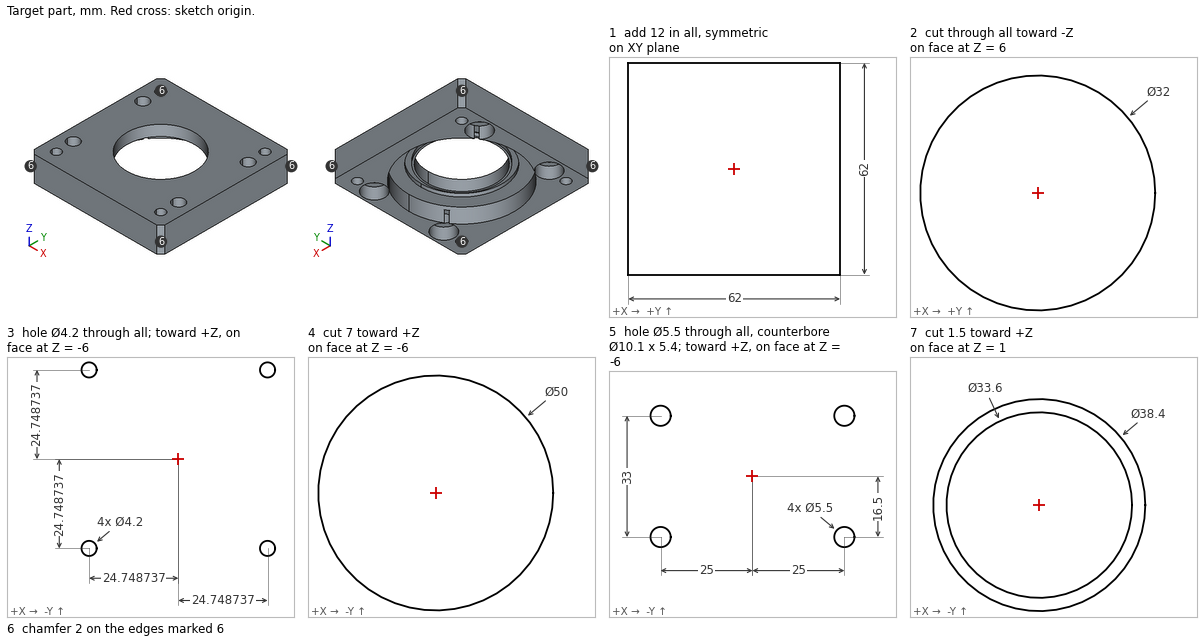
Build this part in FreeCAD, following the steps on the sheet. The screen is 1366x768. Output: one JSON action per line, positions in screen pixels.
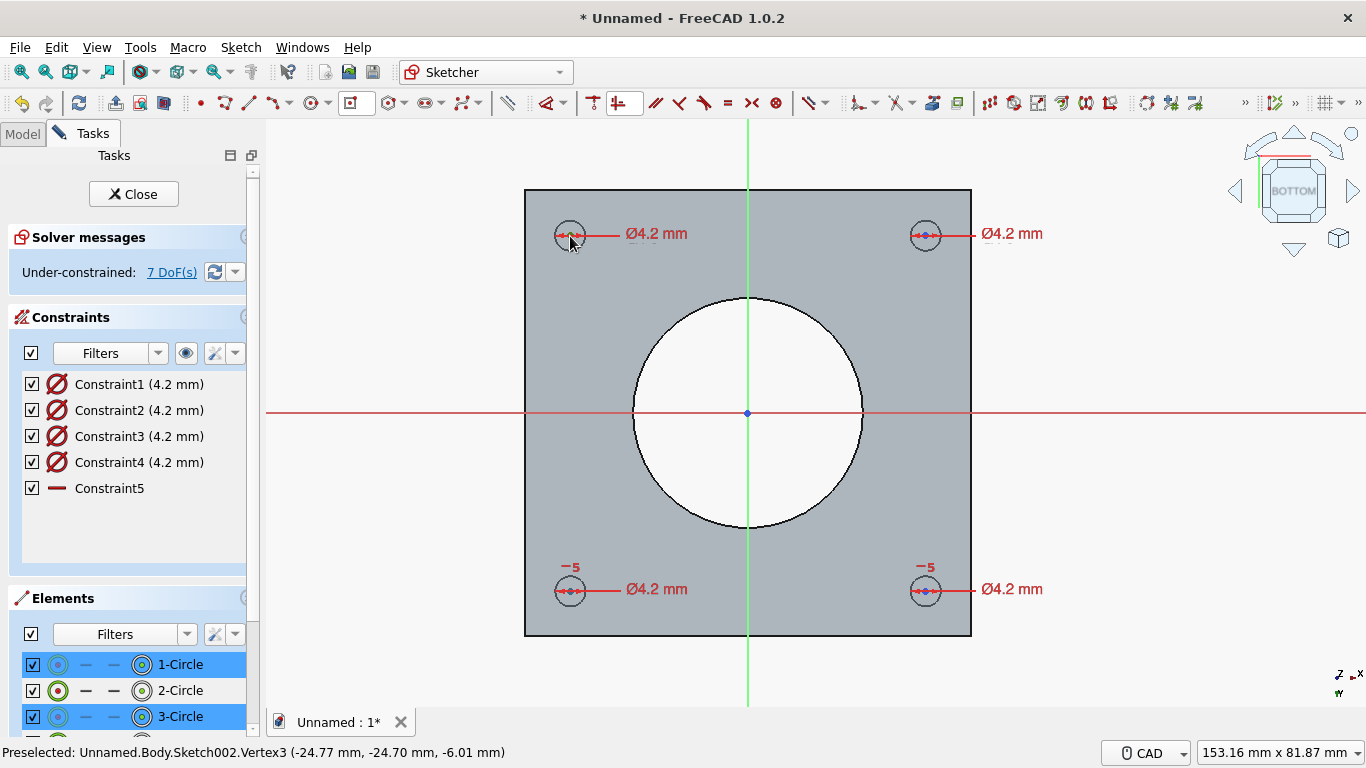
{"action": "left_click", "coordinate": [638, 104]}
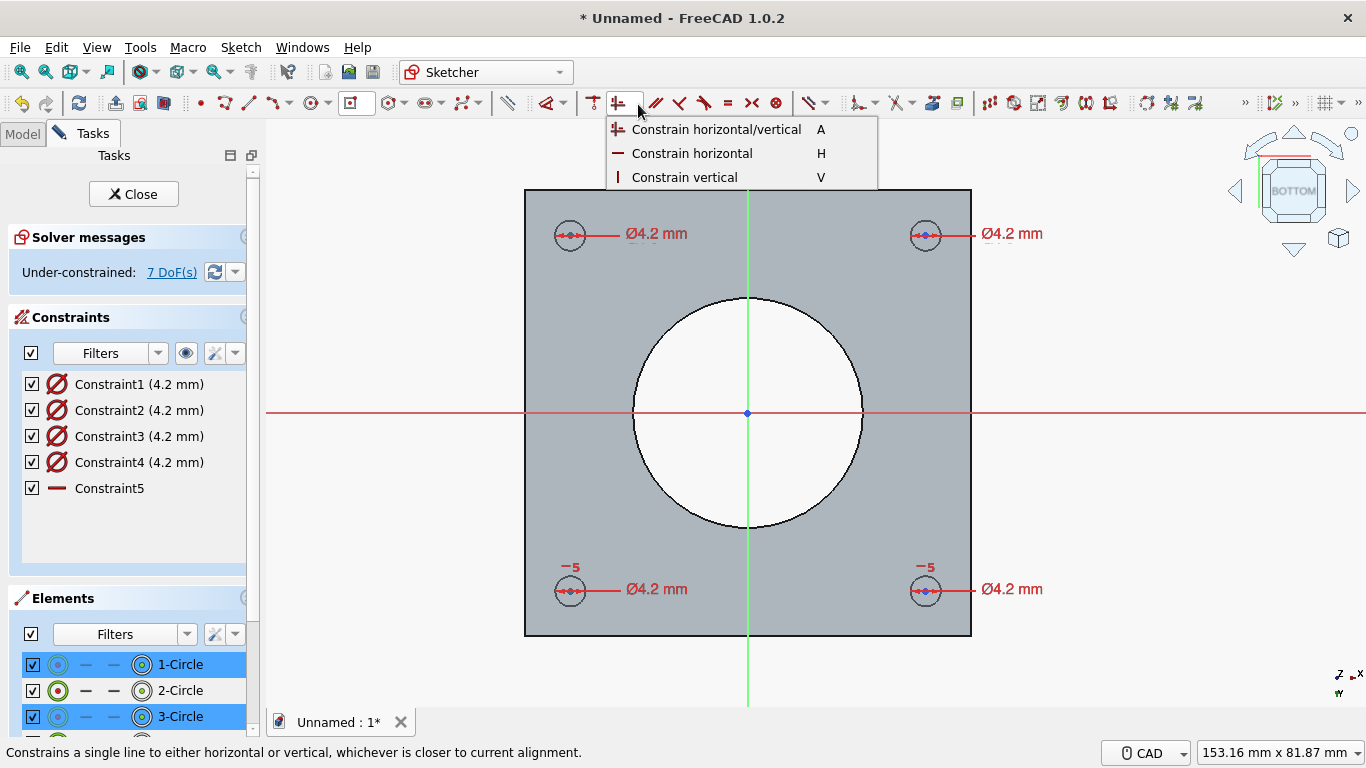
{"action": "left_click", "coordinate": [742, 177]}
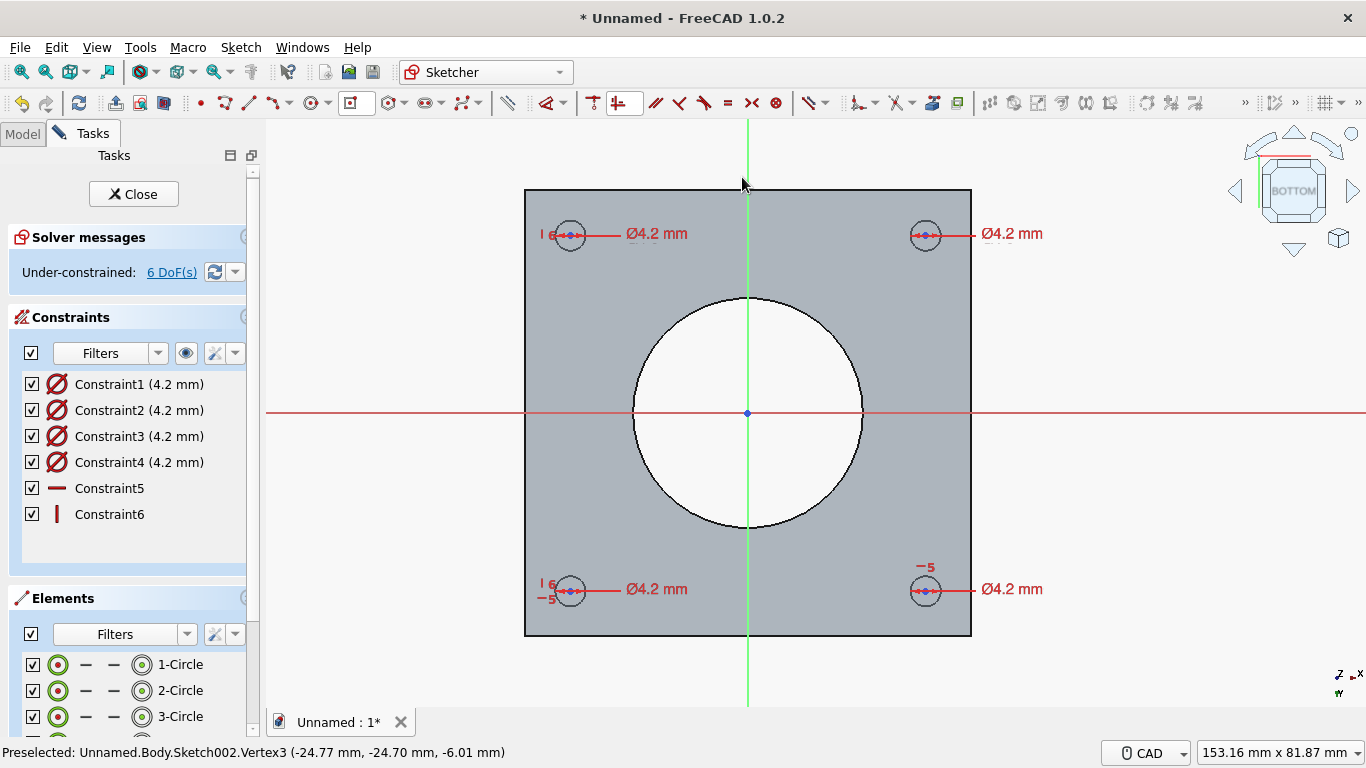
{"action": "left_click", "coordinate": [926, 591]}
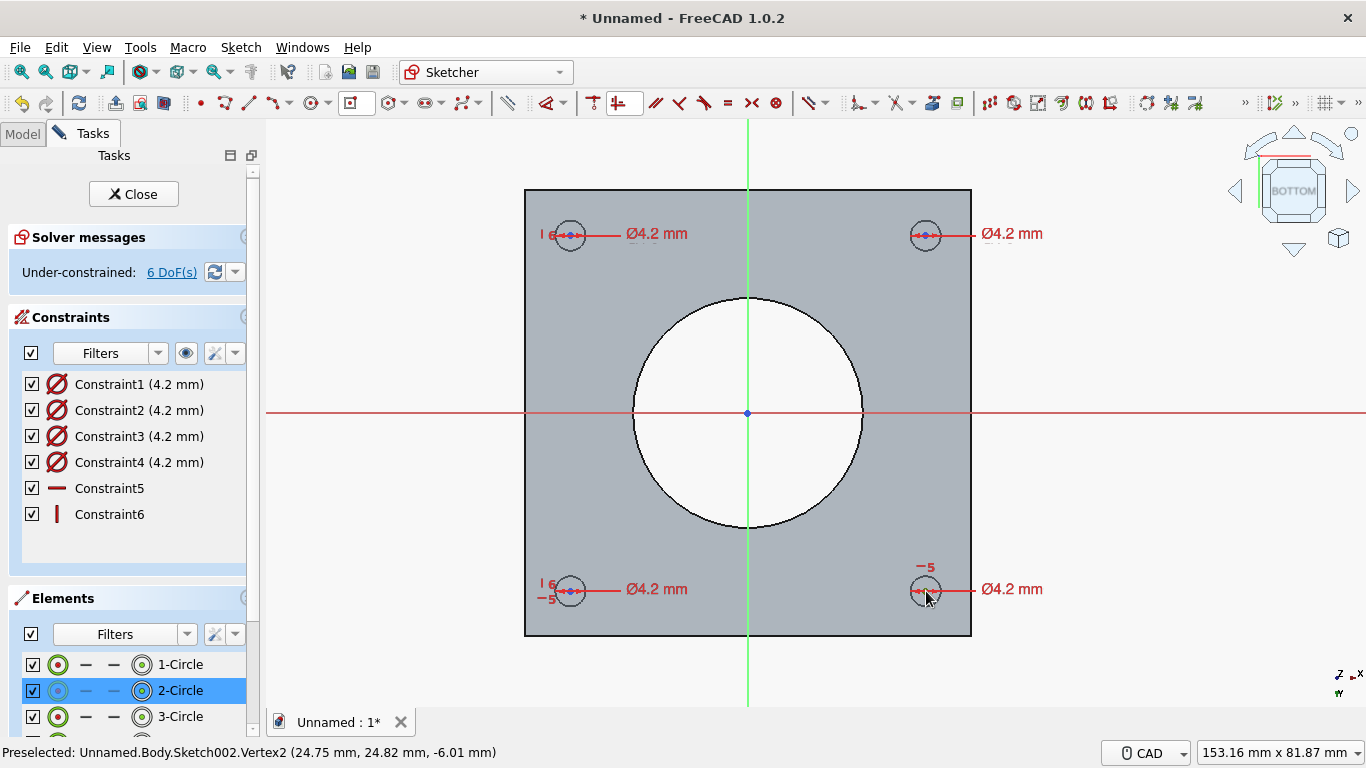
{"action": "left_click", "coordinate": [926, 236]}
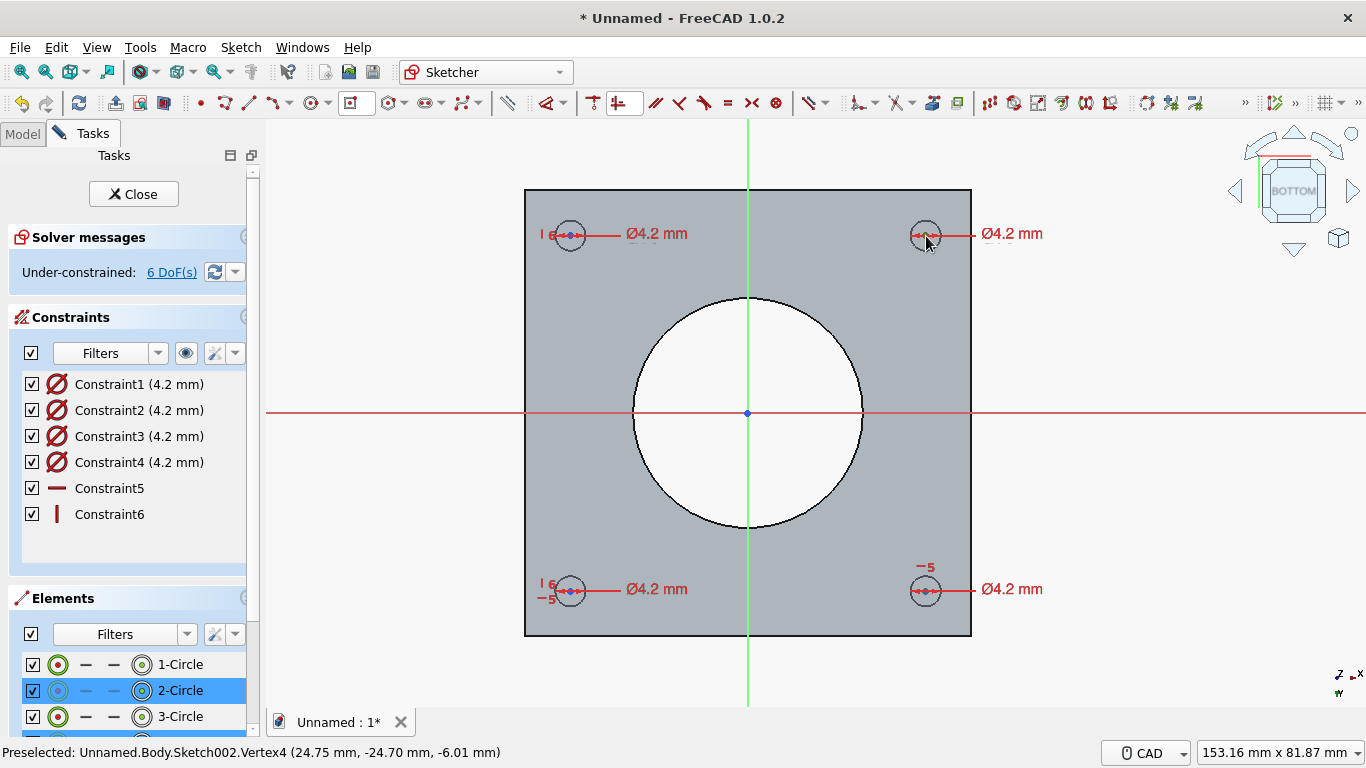
{"action": "left_click", "coordinate": [638, 104]}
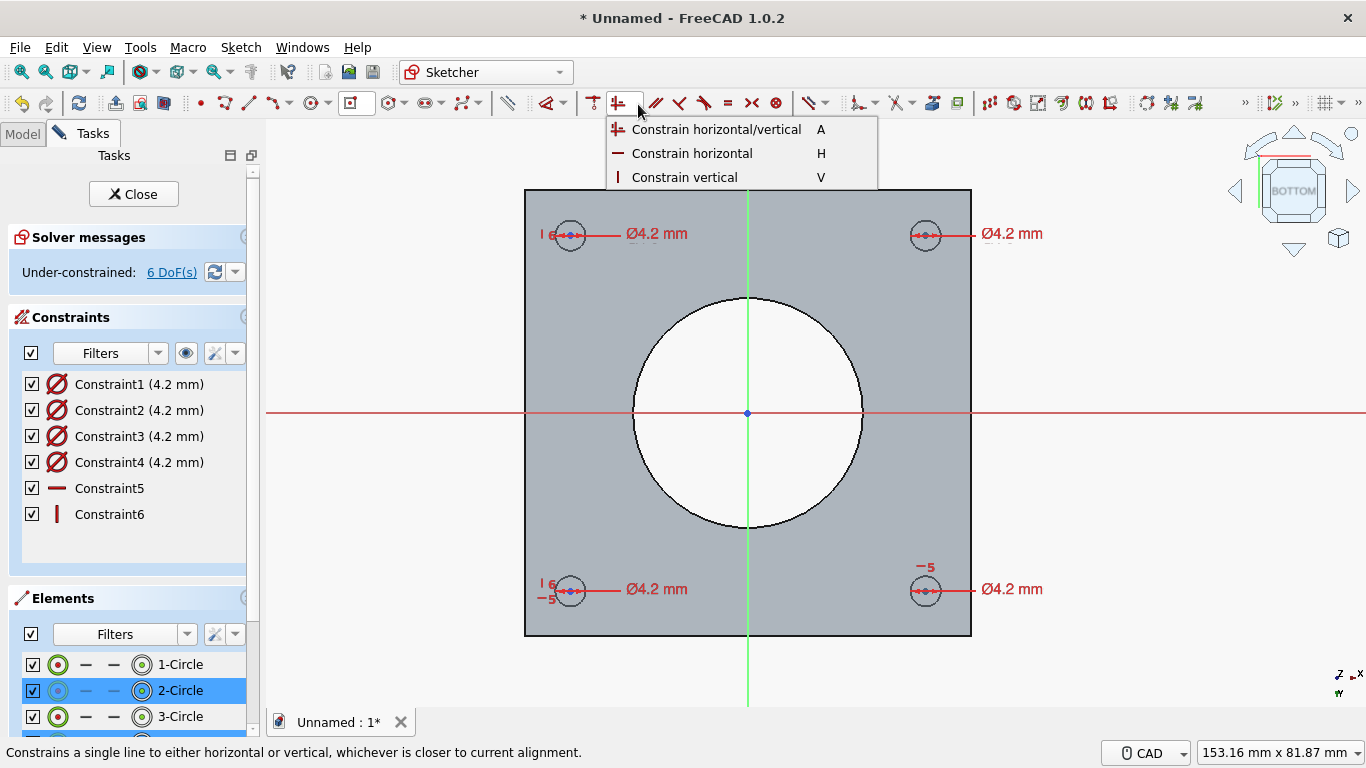
{"action": "left_click", "coordinate": [742, 177]}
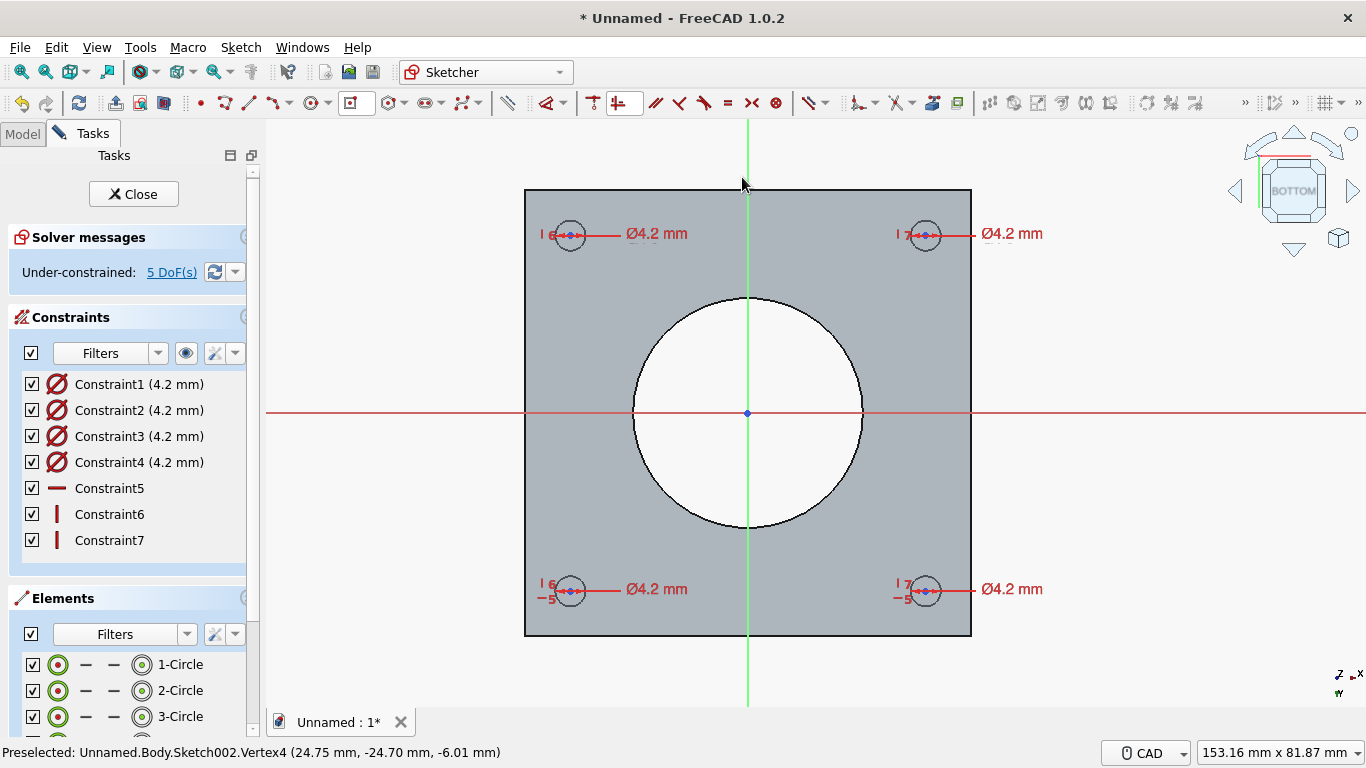
{"action": "left_click", "coordinate": [570, 236]}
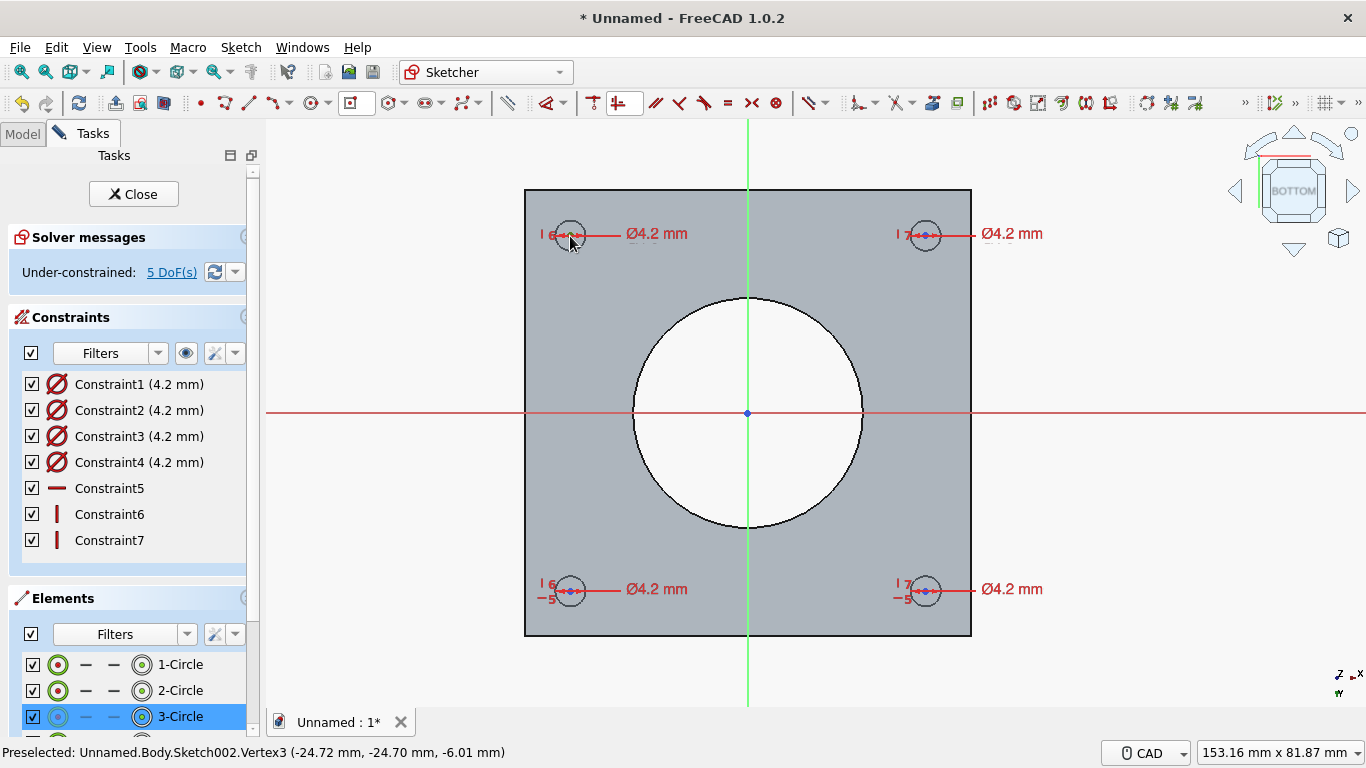
{"action": "left_click", "coordinate": [926, 236]}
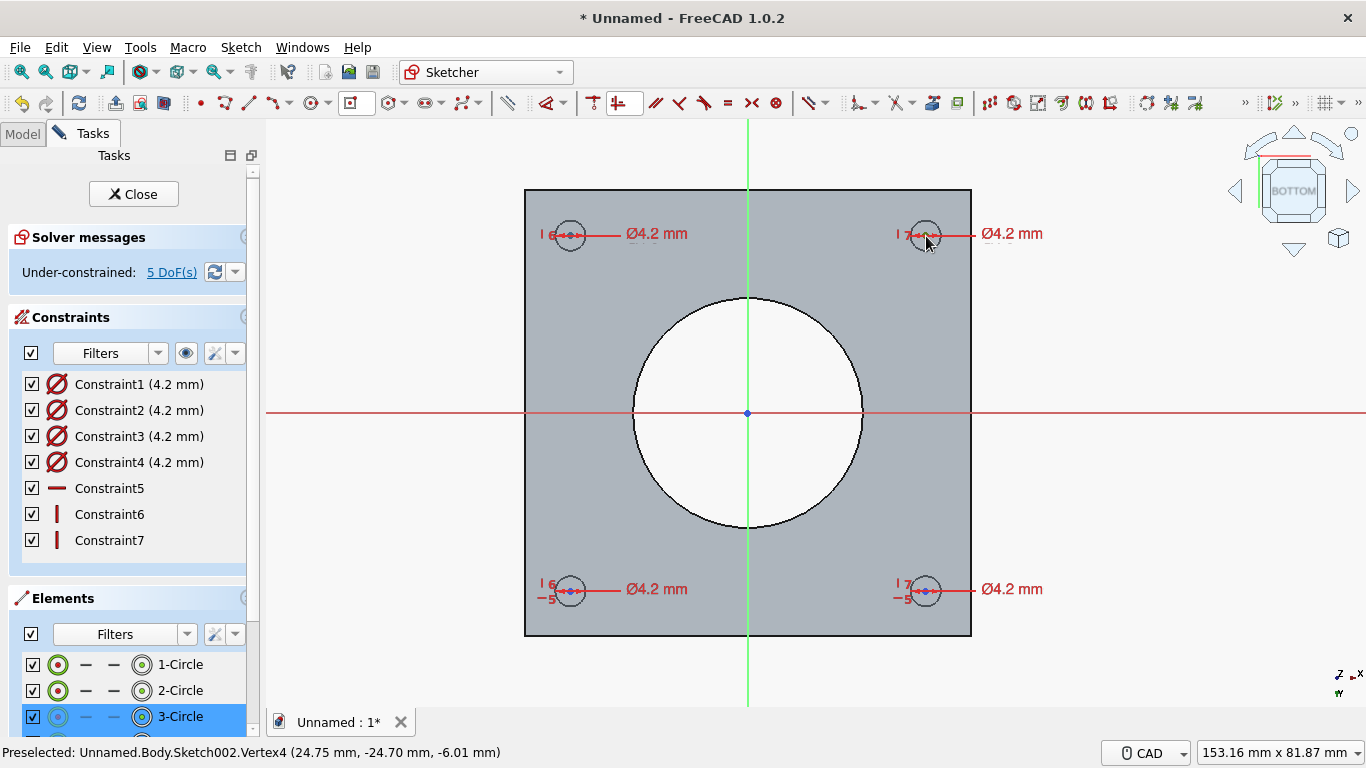
{"action": "left_click", "coordinate": [638, 104]}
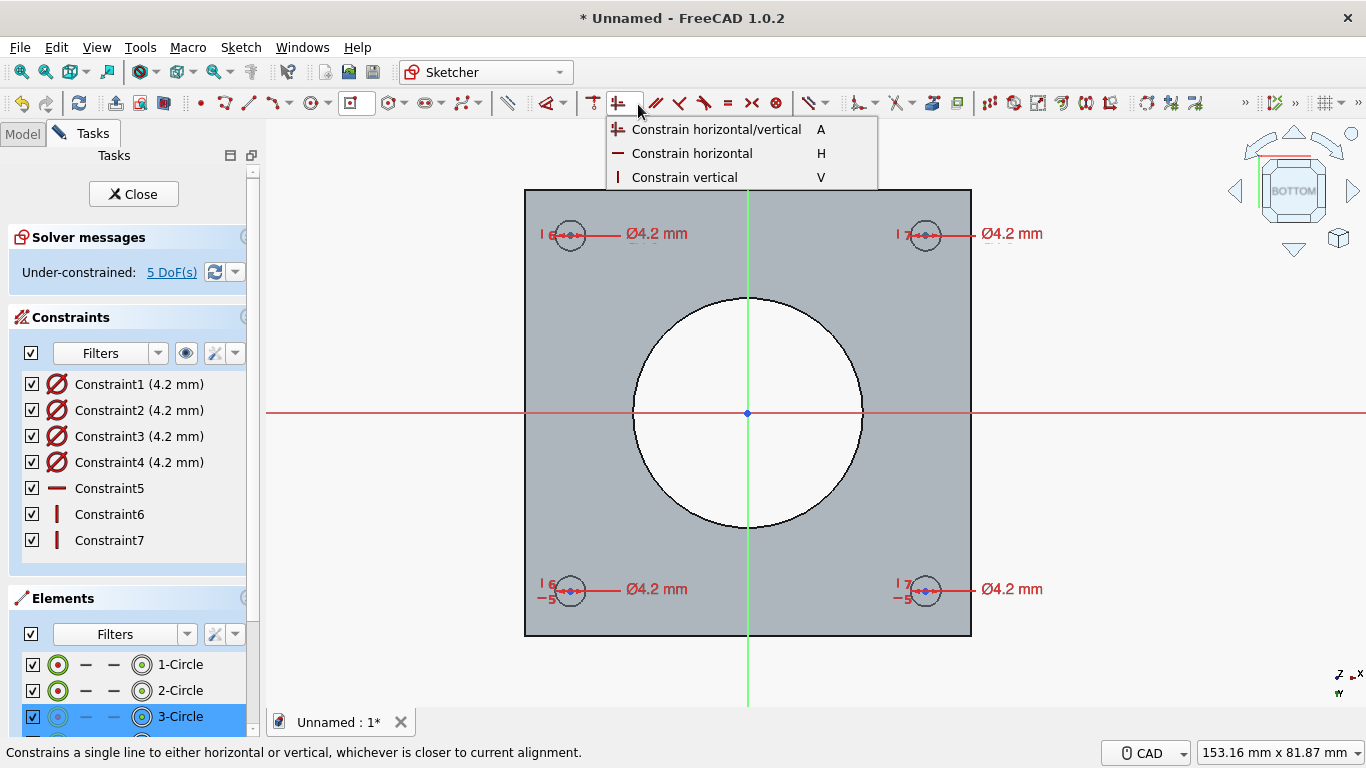
{"action": "left_click", "coordinate": [742, 153]}